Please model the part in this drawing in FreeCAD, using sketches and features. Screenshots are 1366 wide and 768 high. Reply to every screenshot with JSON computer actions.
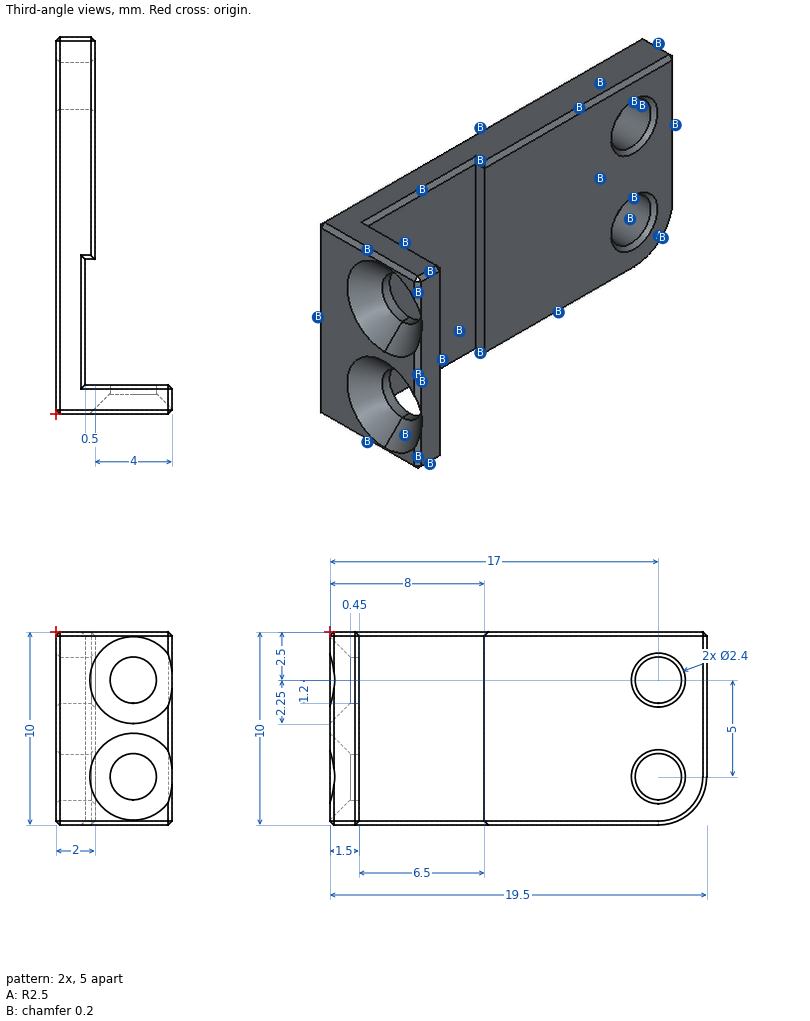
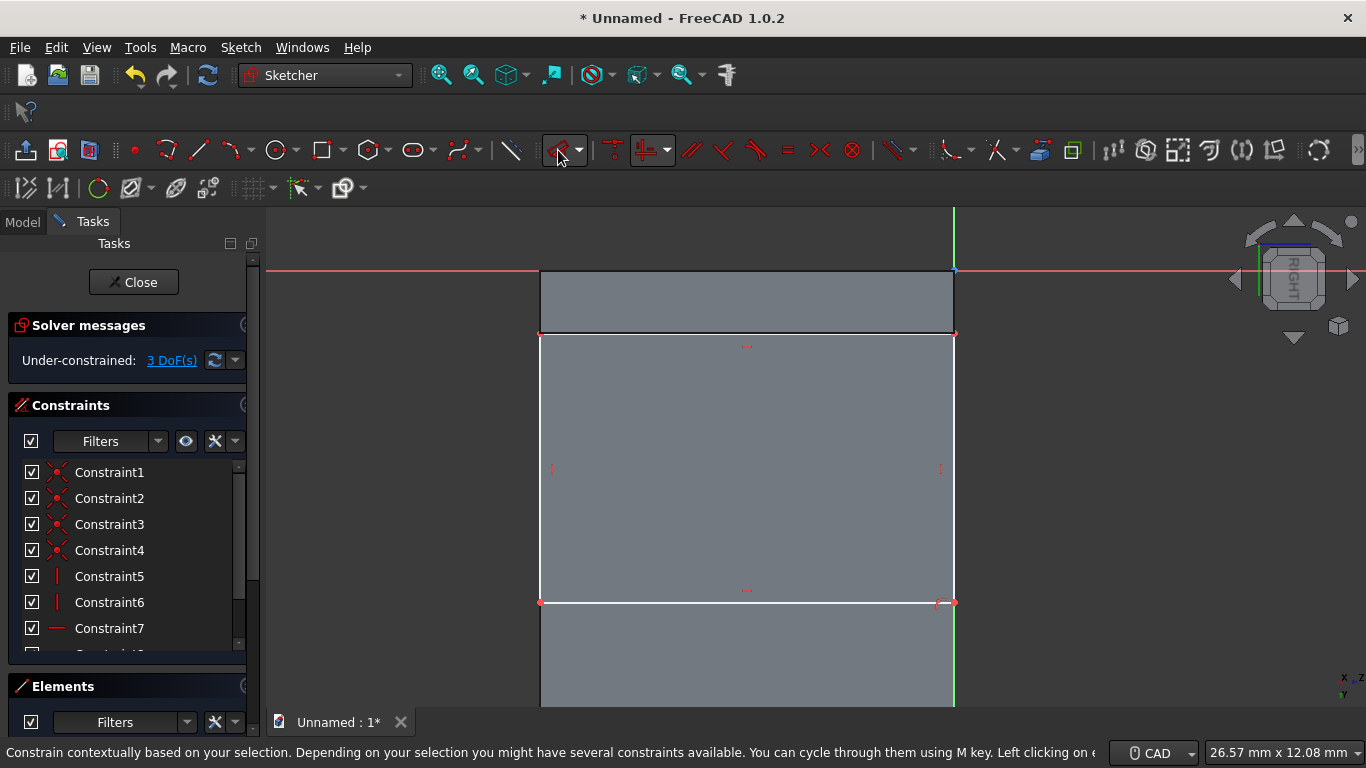
{"action": "left_click", "coordinate": [664, 603]}
{"action": "left_click", "coordinate": [747, 637]}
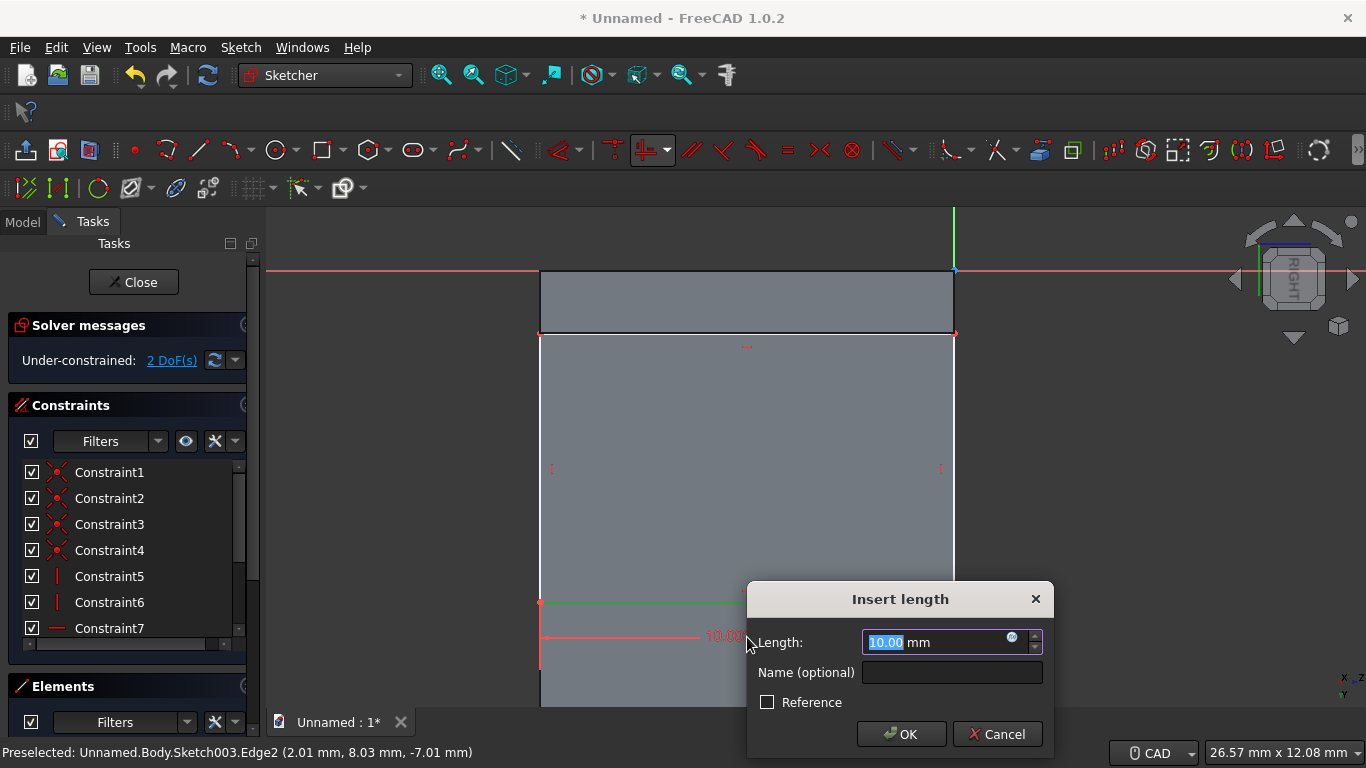
{"action": "type", "text": "10"}
{"action": "key", "text": "Return"}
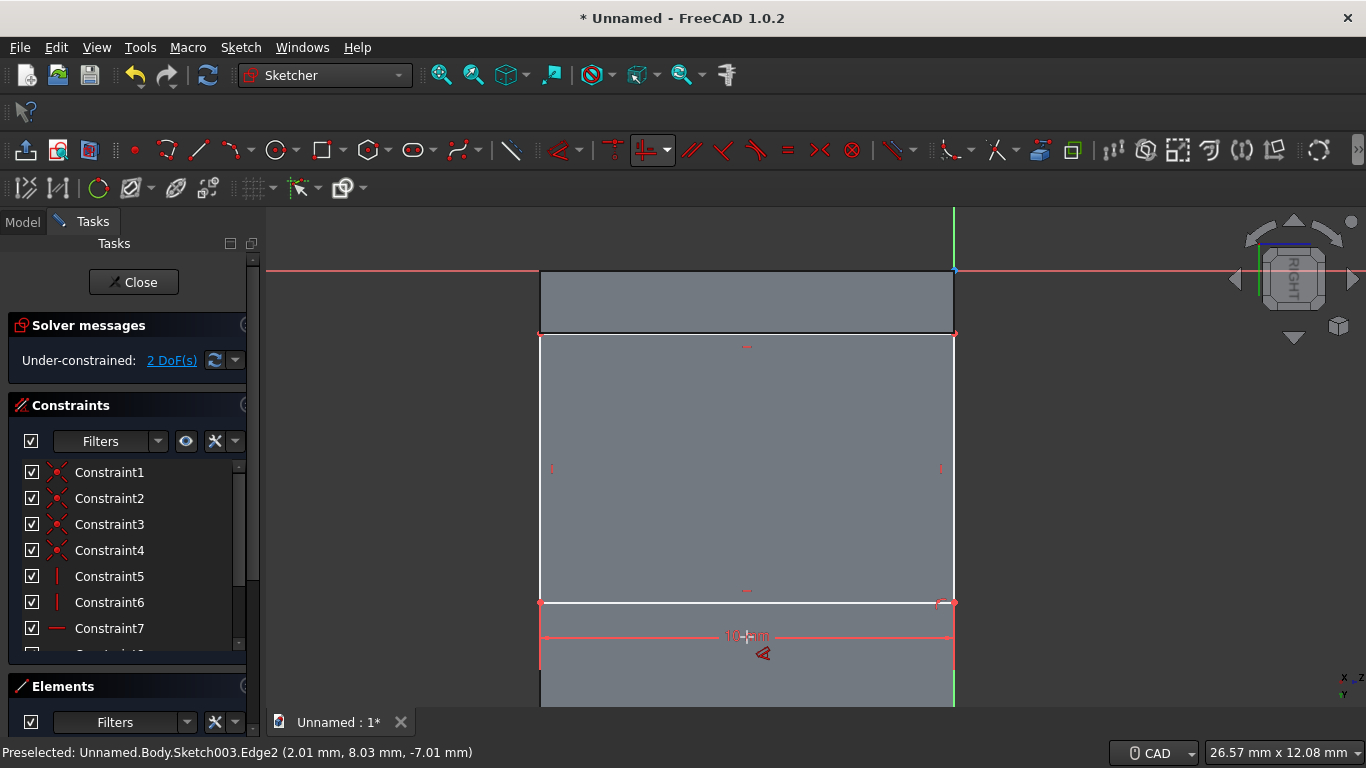
{"action": "left_click", "coordinate": [540, 603]}
{"action": "left_click", "coordinate": [988, 437]}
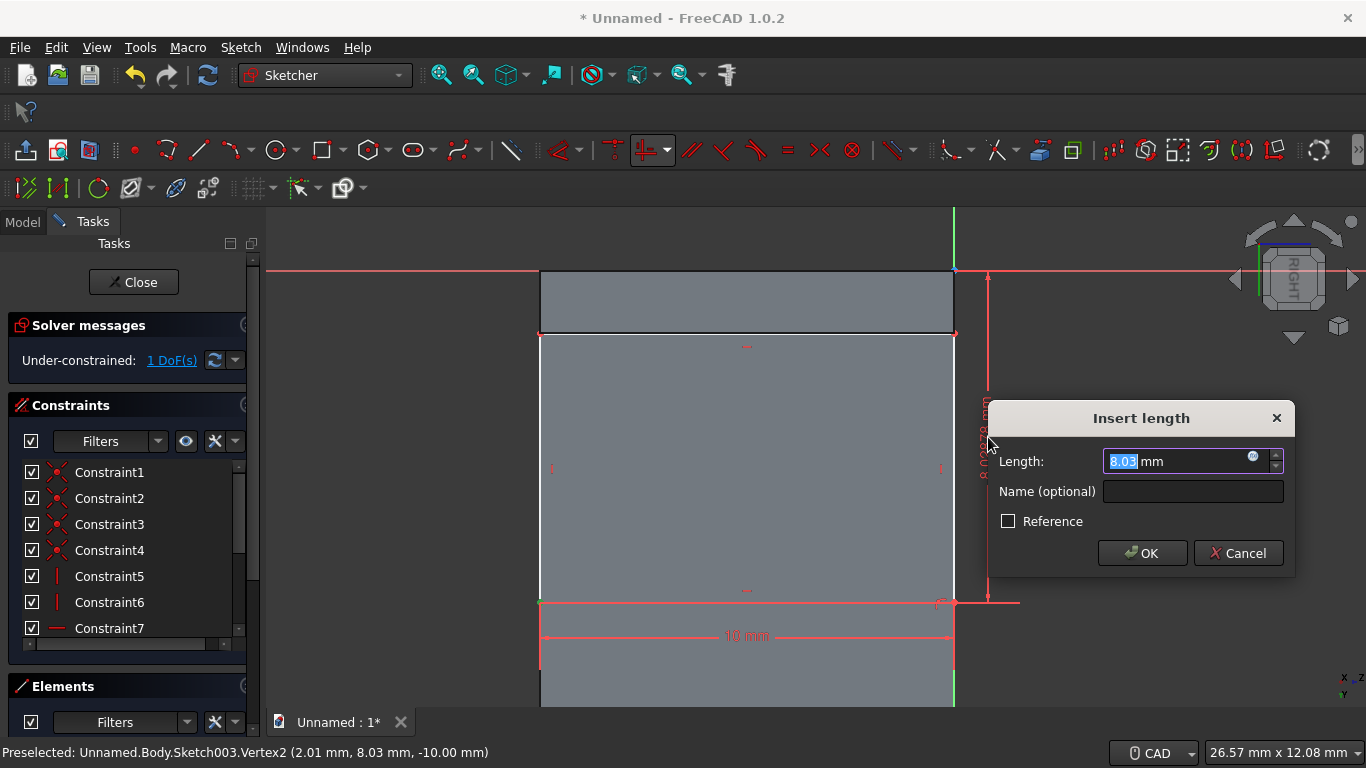
{"action": "type", "text": "8"}
{"action": "key", "text": "Return"}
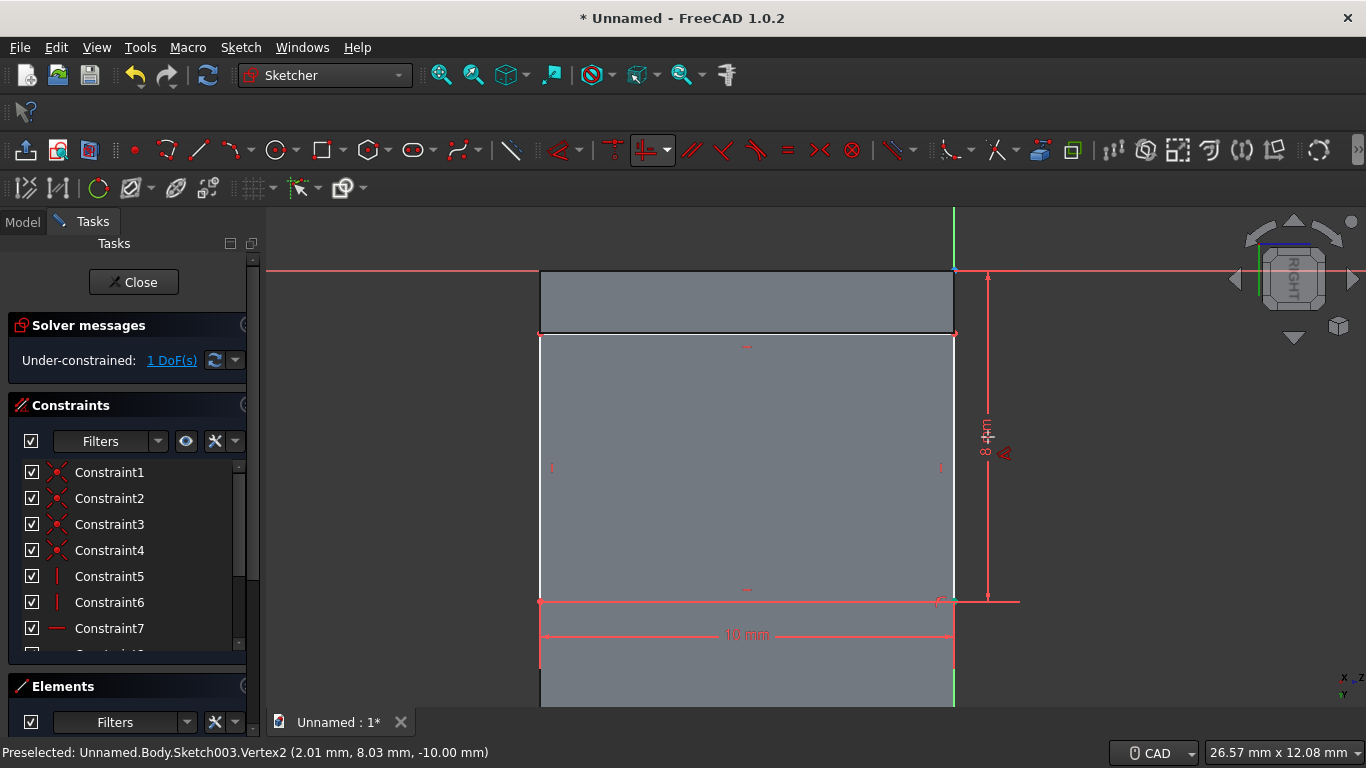
{"action": "left_click", "coordinate": [540, 414]}
{"action": "left_click", "coordinate": [506, 468]}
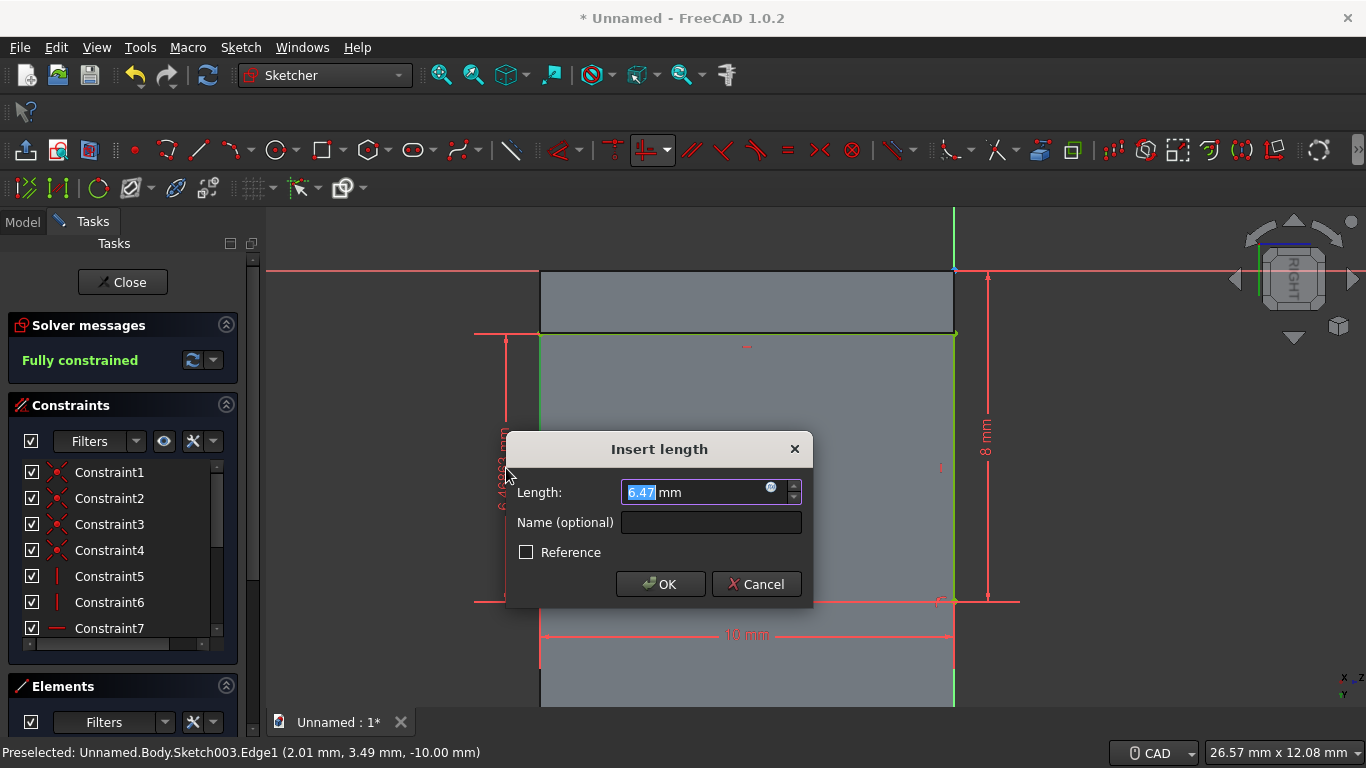
{"action": "type", "text": "6.5"}
{"action": "key", "text": "Return"}
{"action": "key", "text": "Escape"}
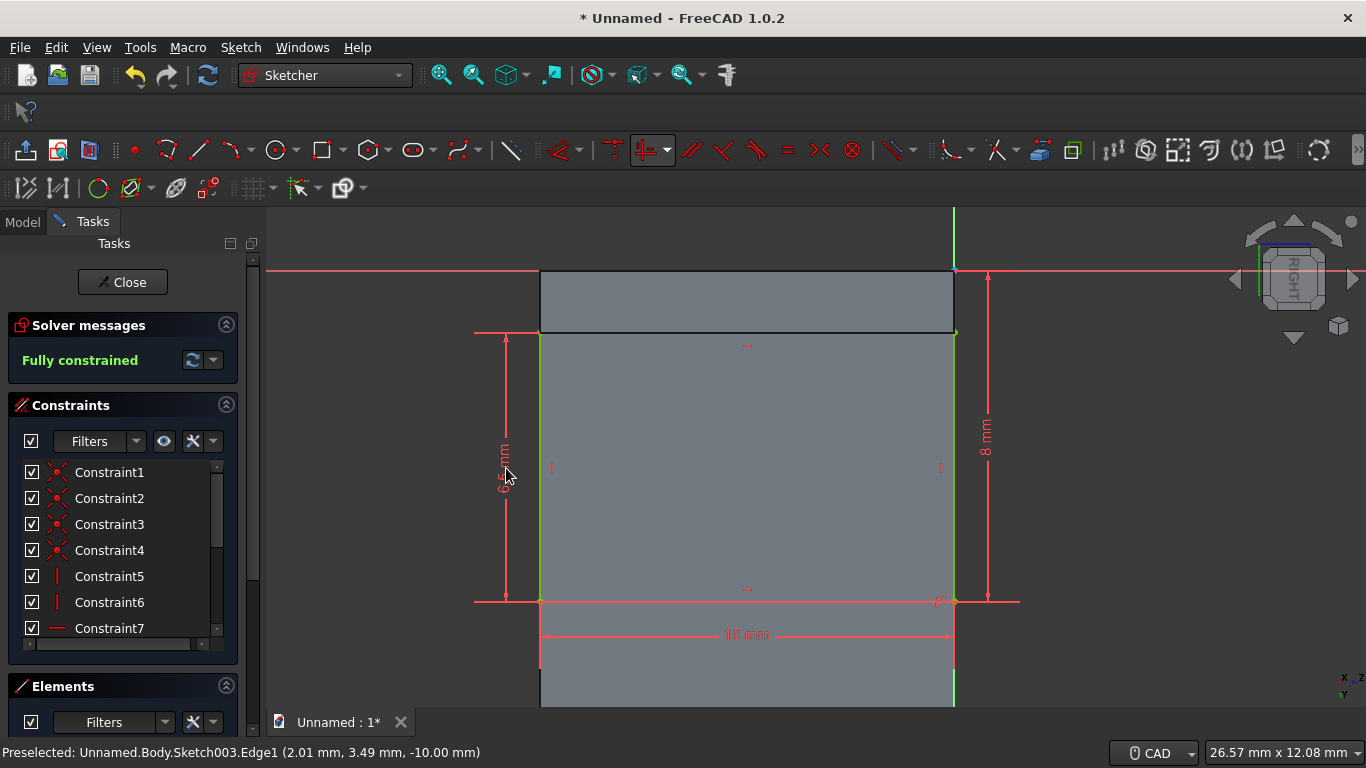
{"action": "left_click", "coordinate": [123, 282]}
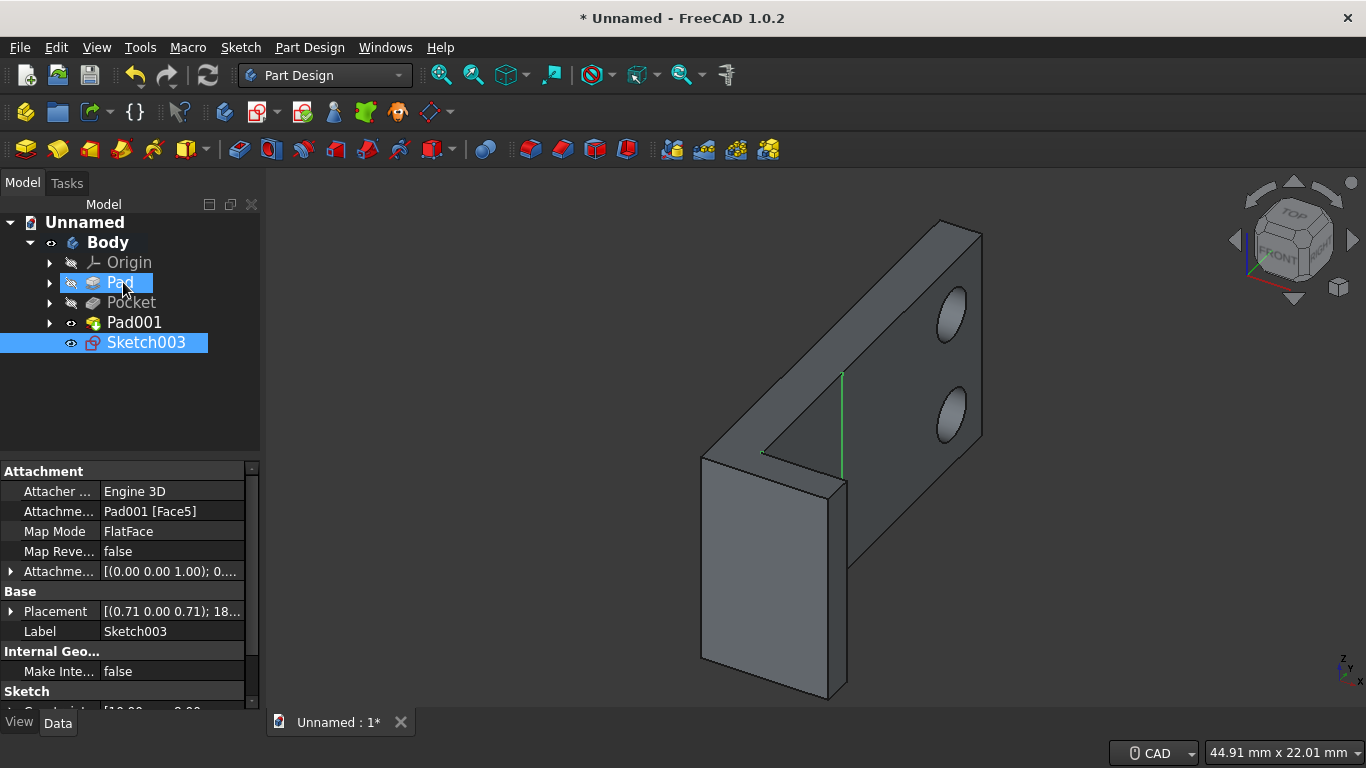
{"action": "left_click", "coordinate": [240, 150]}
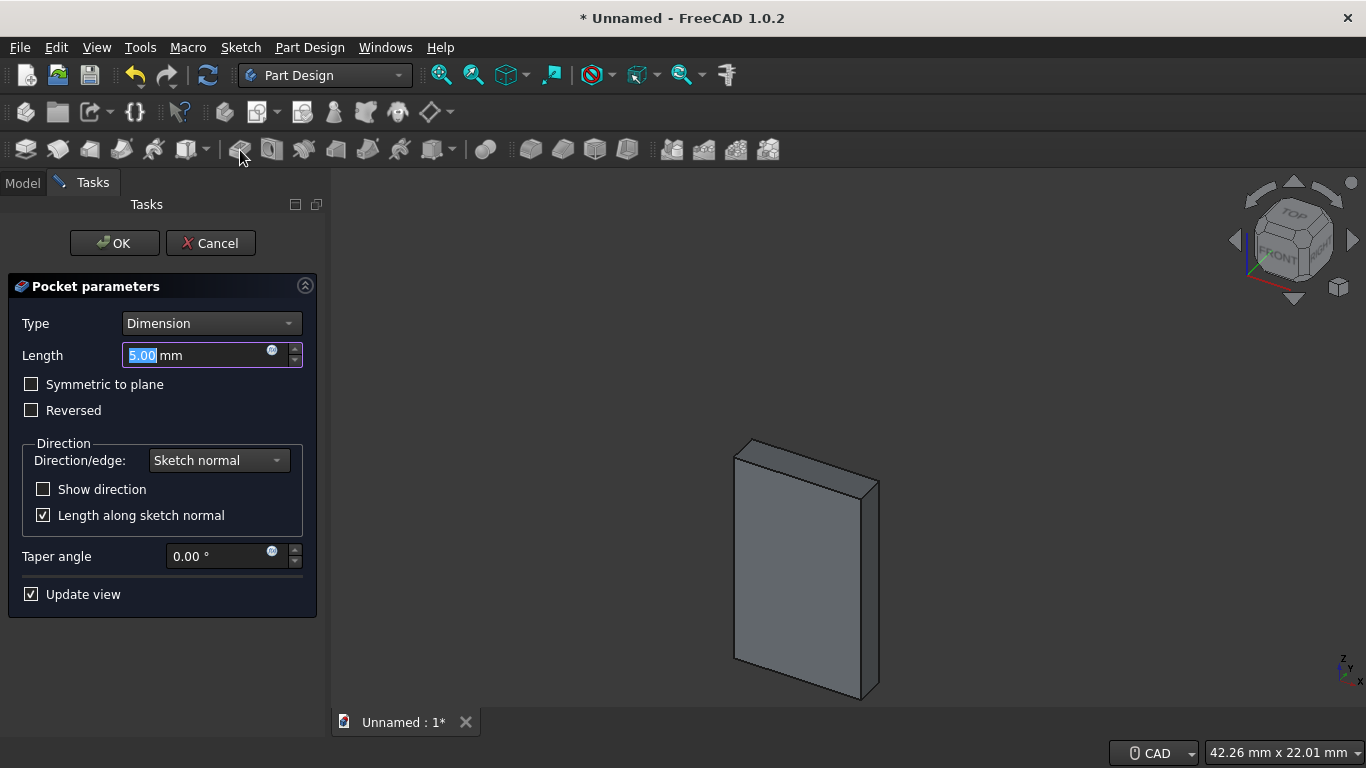
{"action": "type", "text": "0.5"}
{"action": "key", "text": "Tab"}